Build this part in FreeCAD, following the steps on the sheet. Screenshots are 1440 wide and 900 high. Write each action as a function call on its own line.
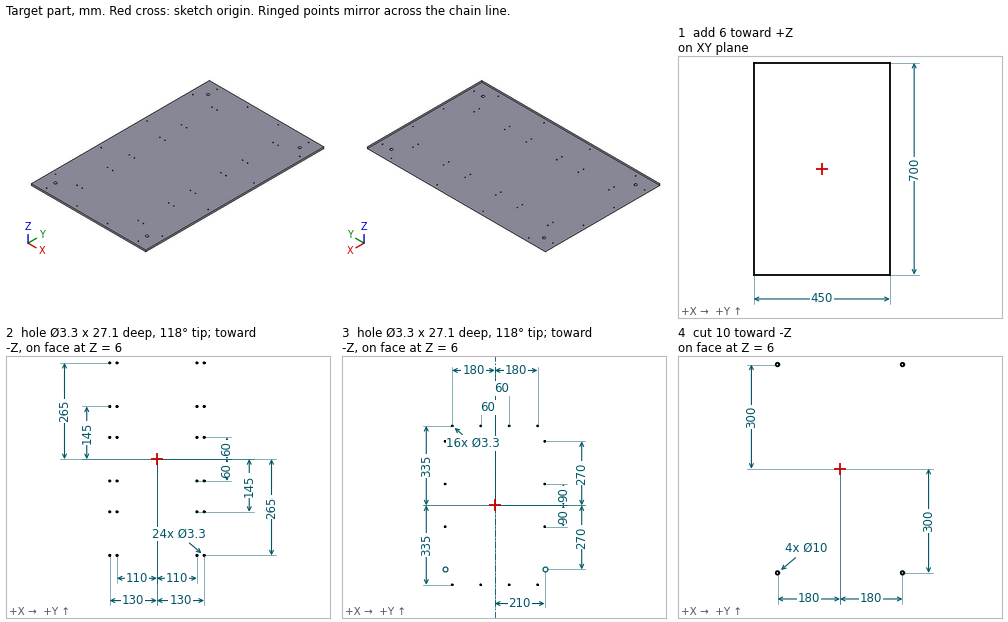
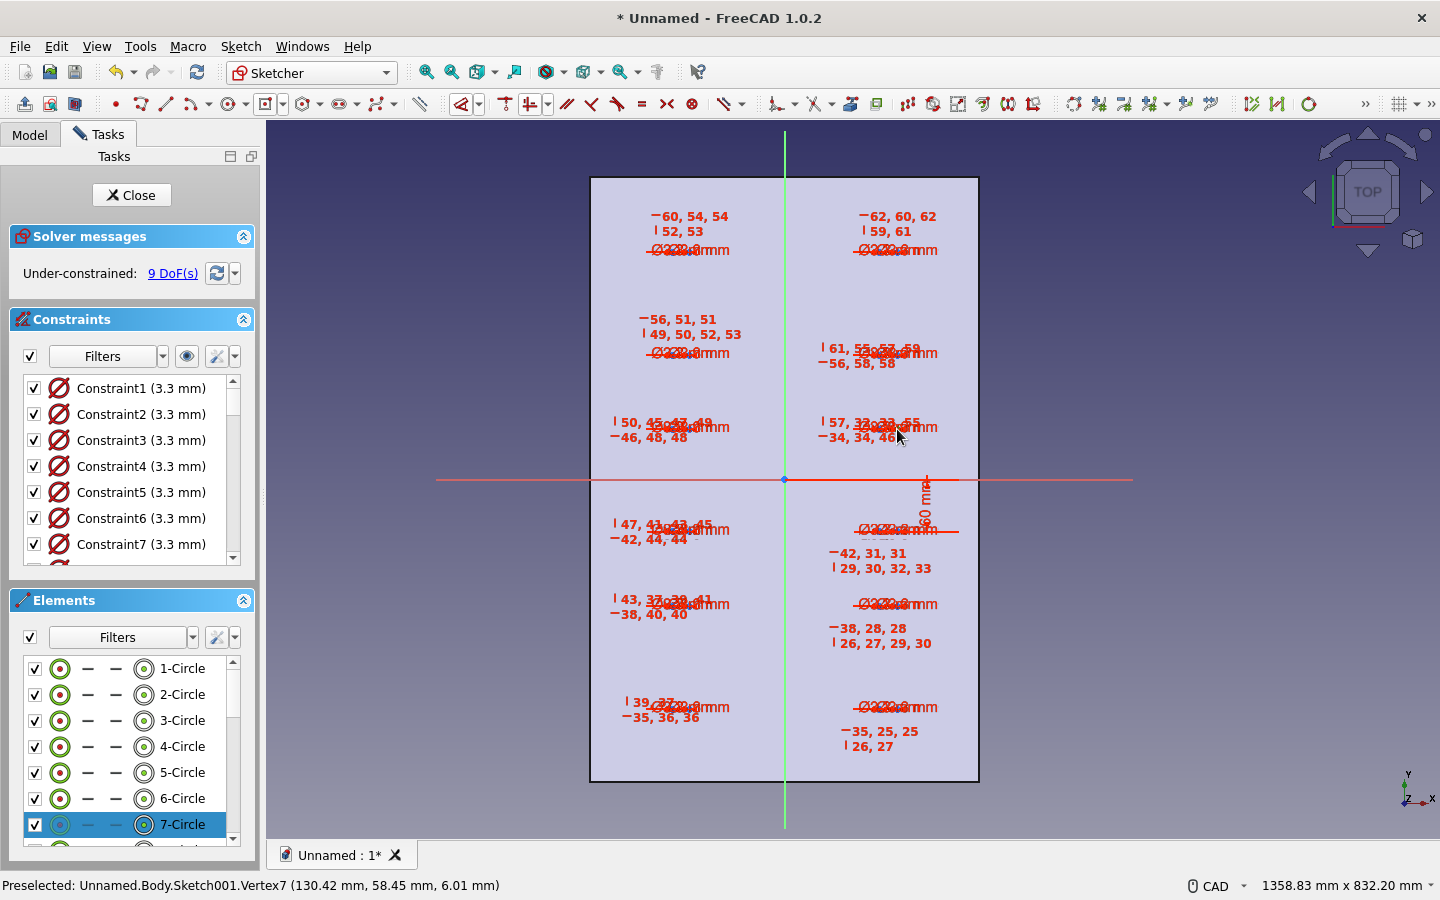
click(478, 104)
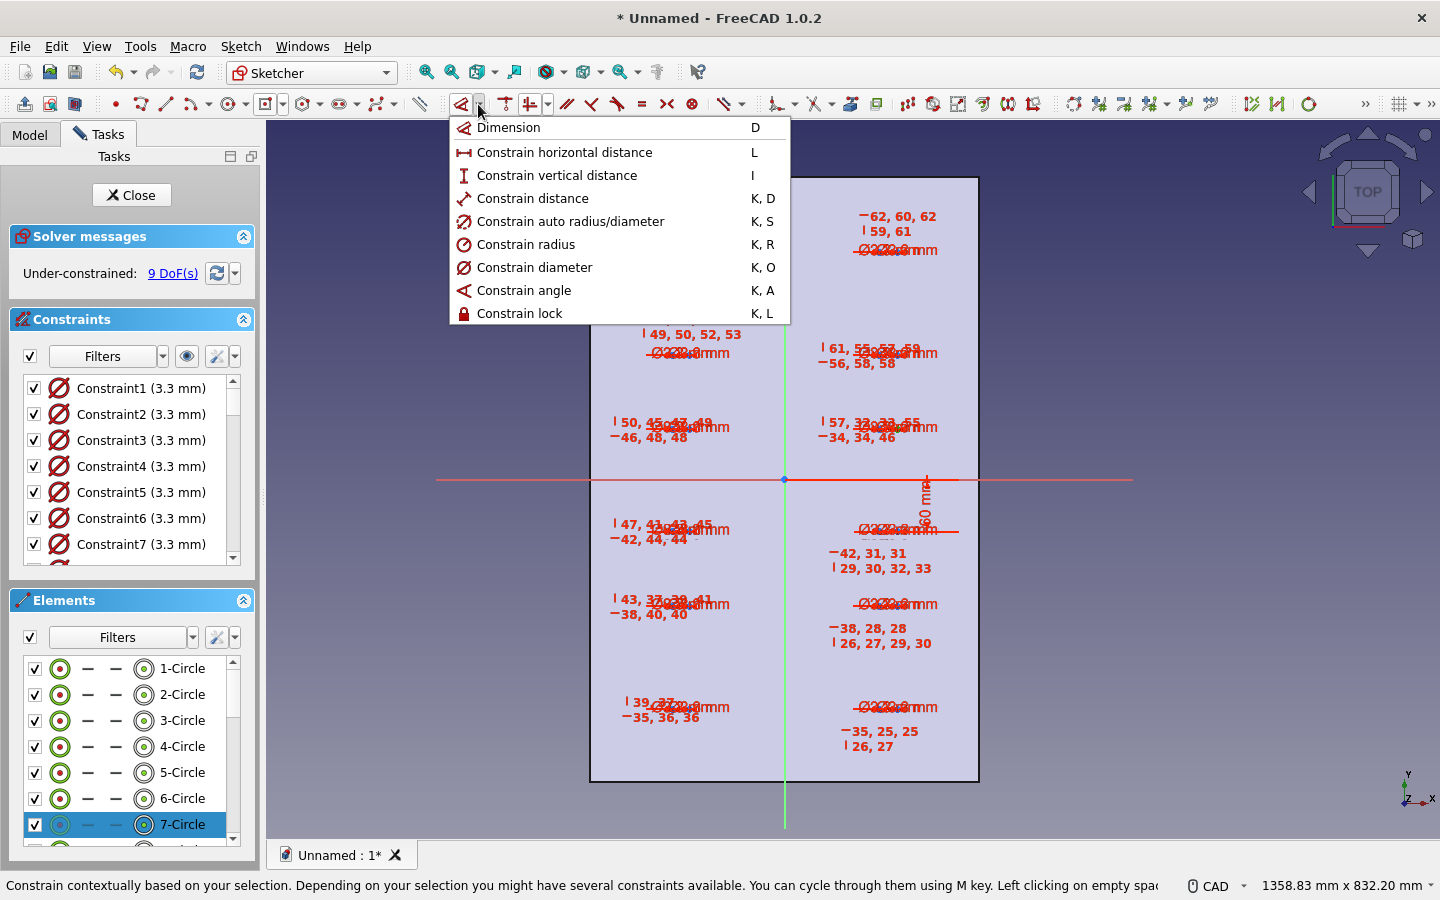
click(620, 176)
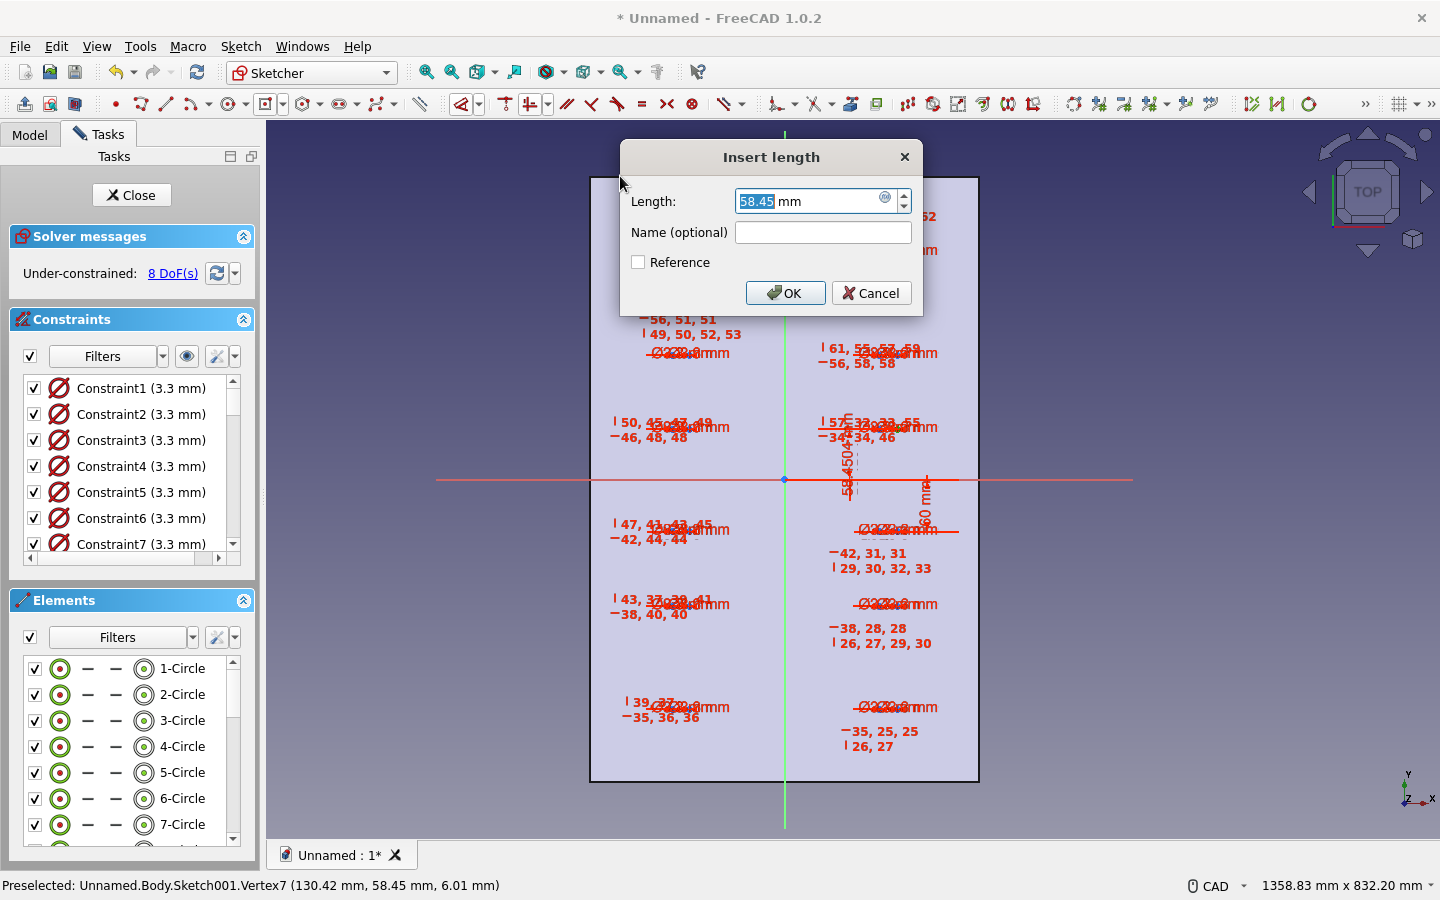
text(60)
key(Return)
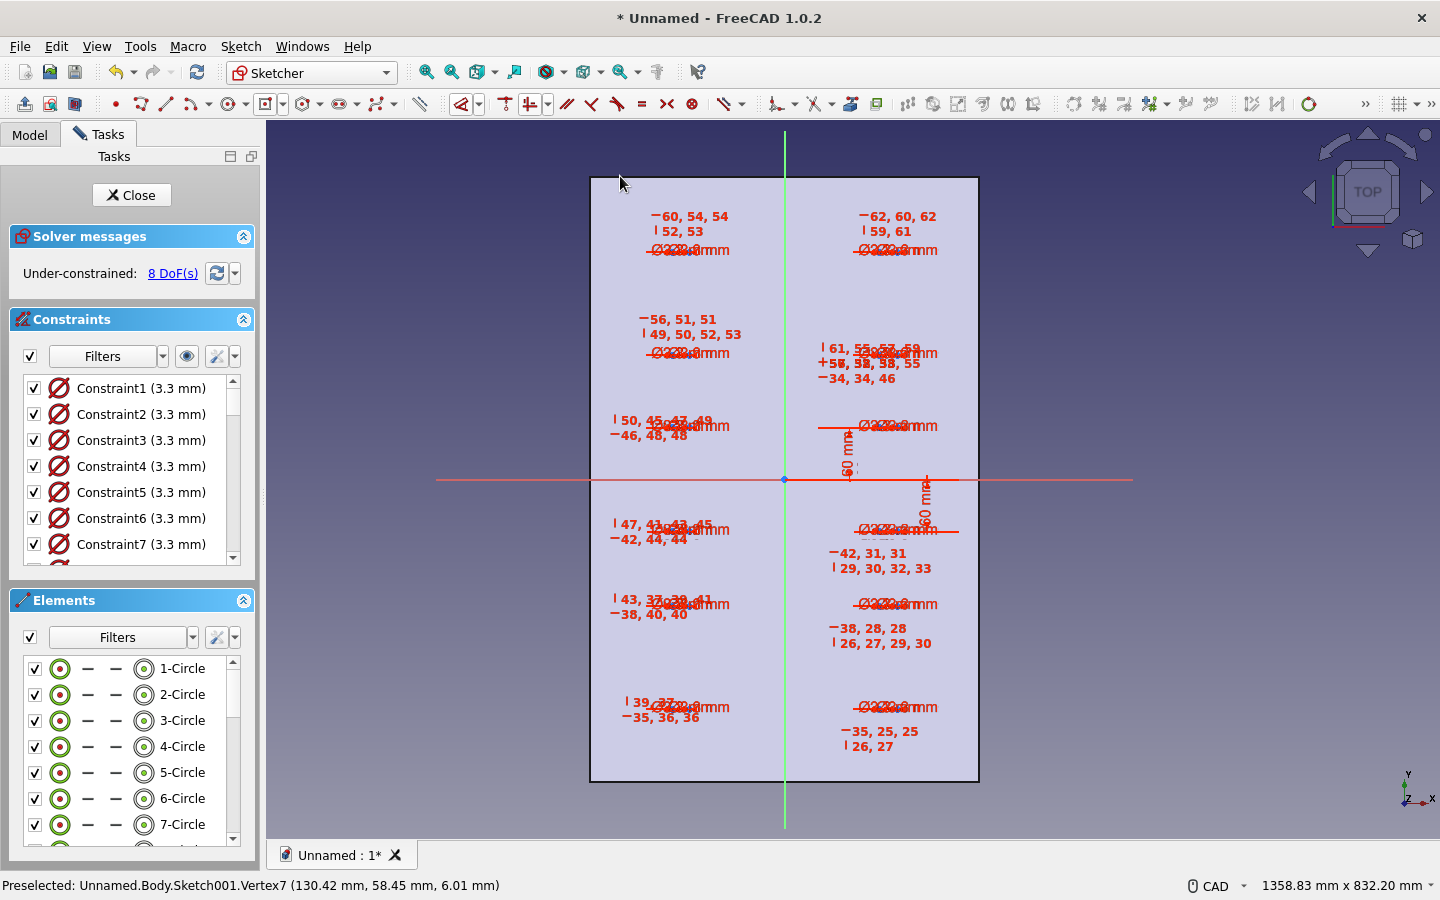
click(897, 709)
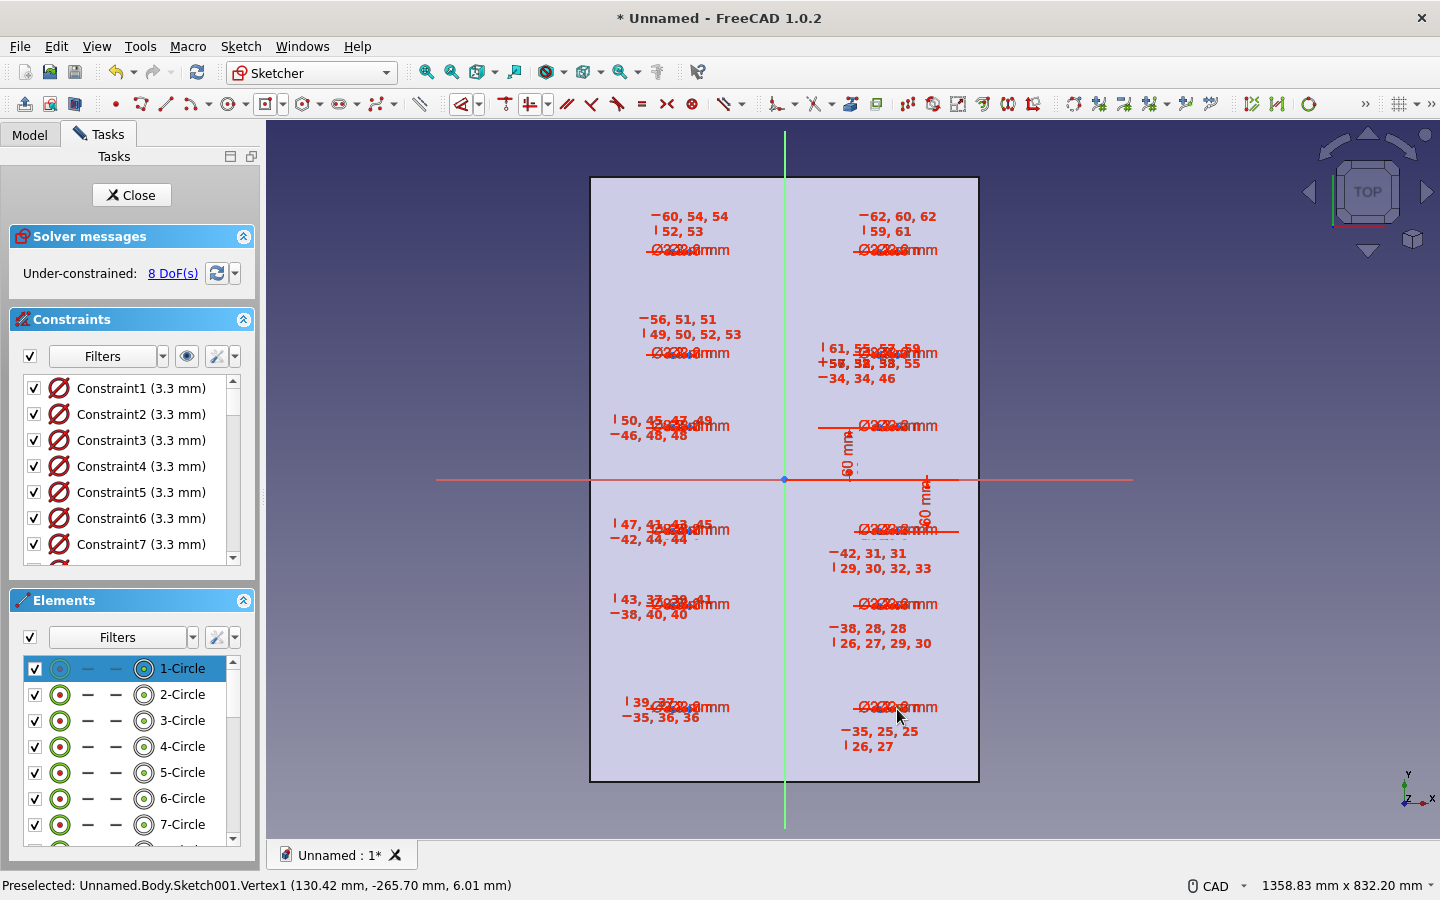
key(l)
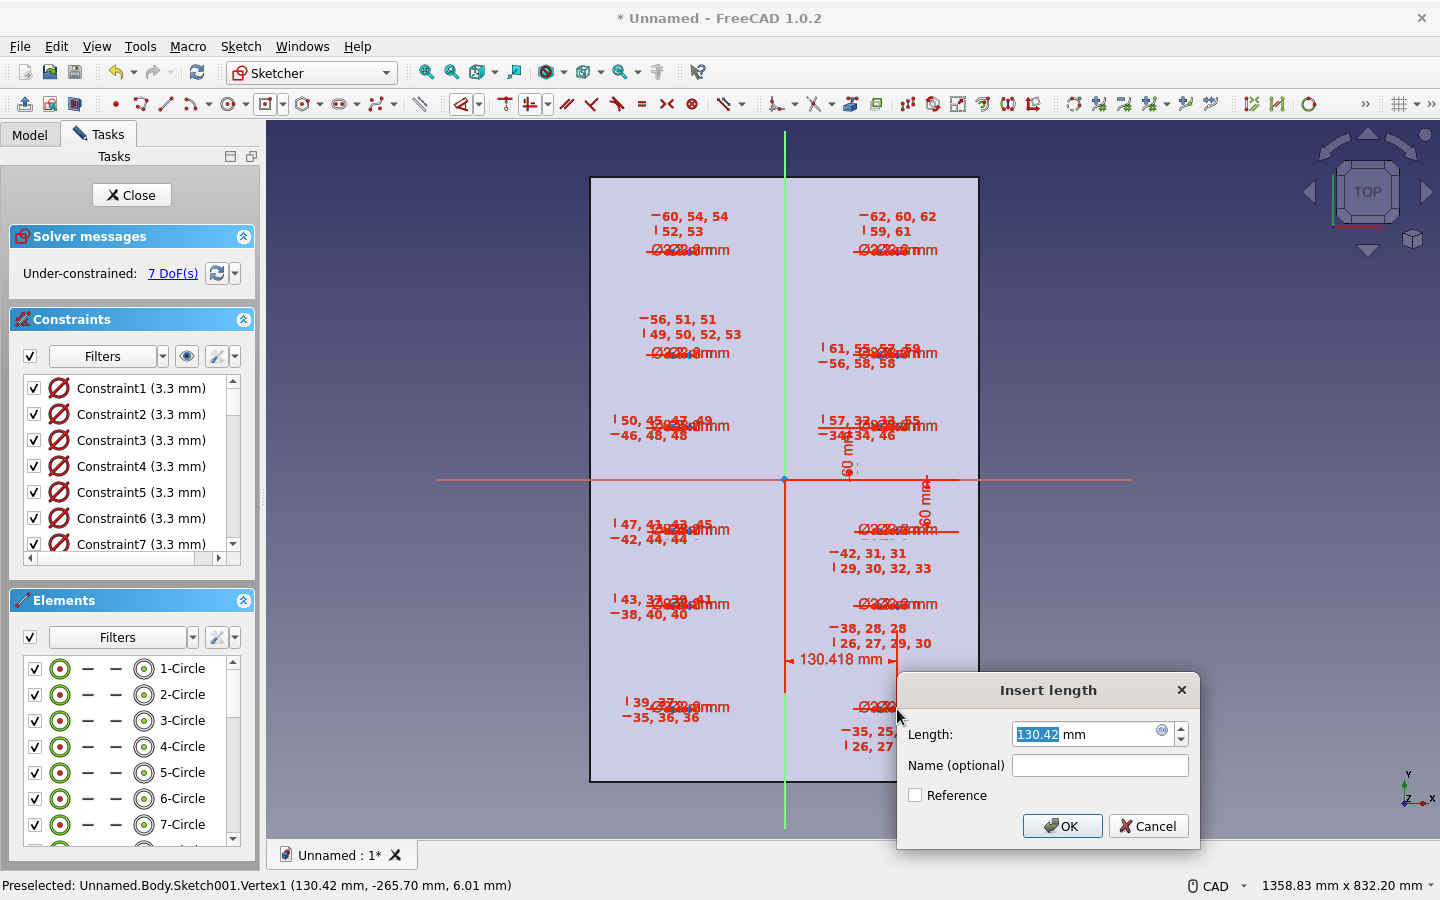
text(130)
key(Return)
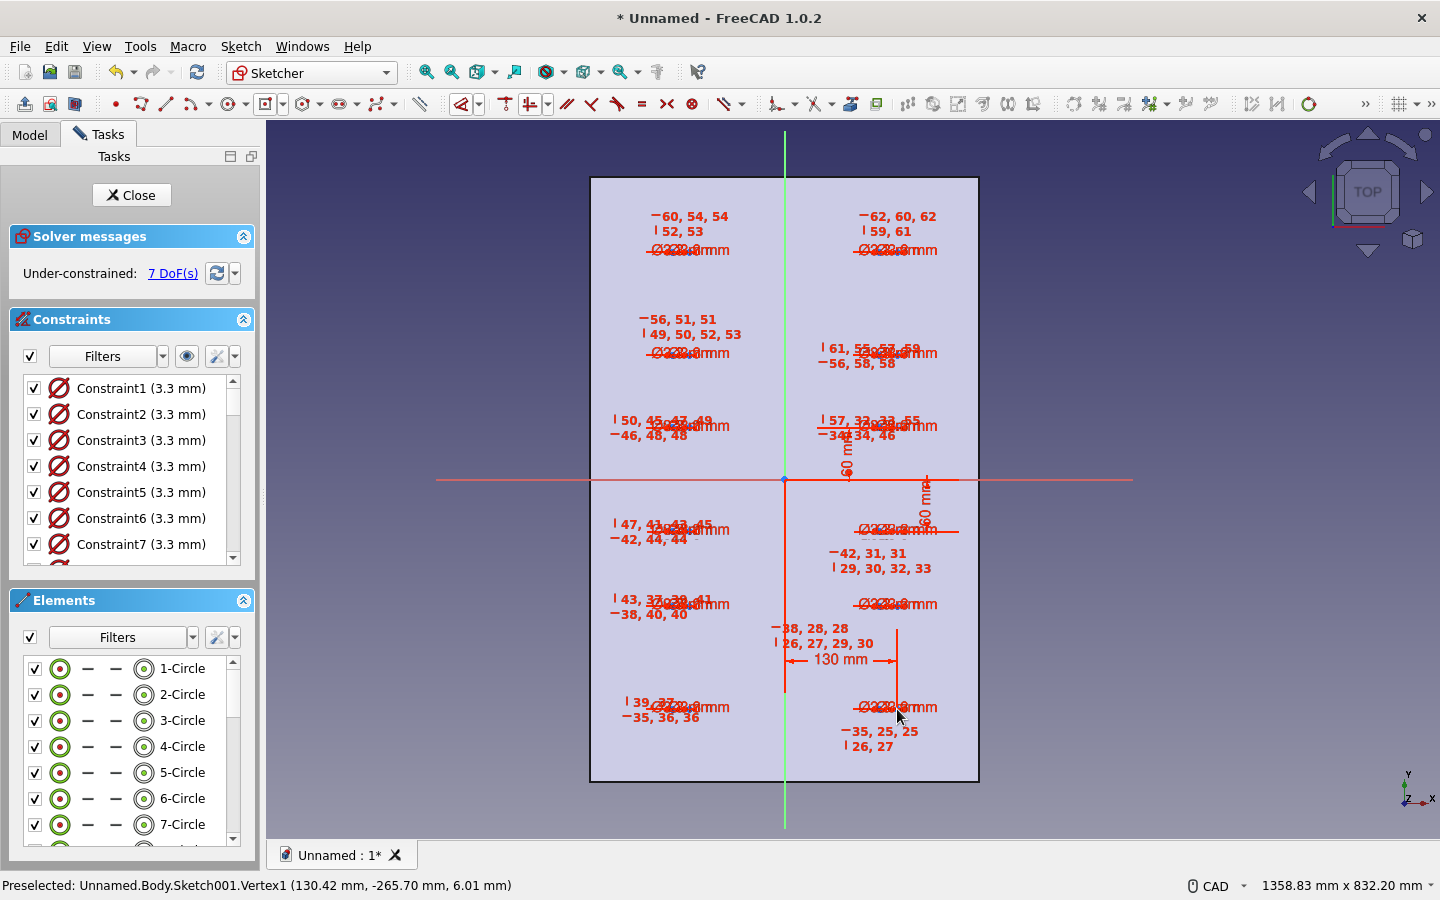
click(897, 709)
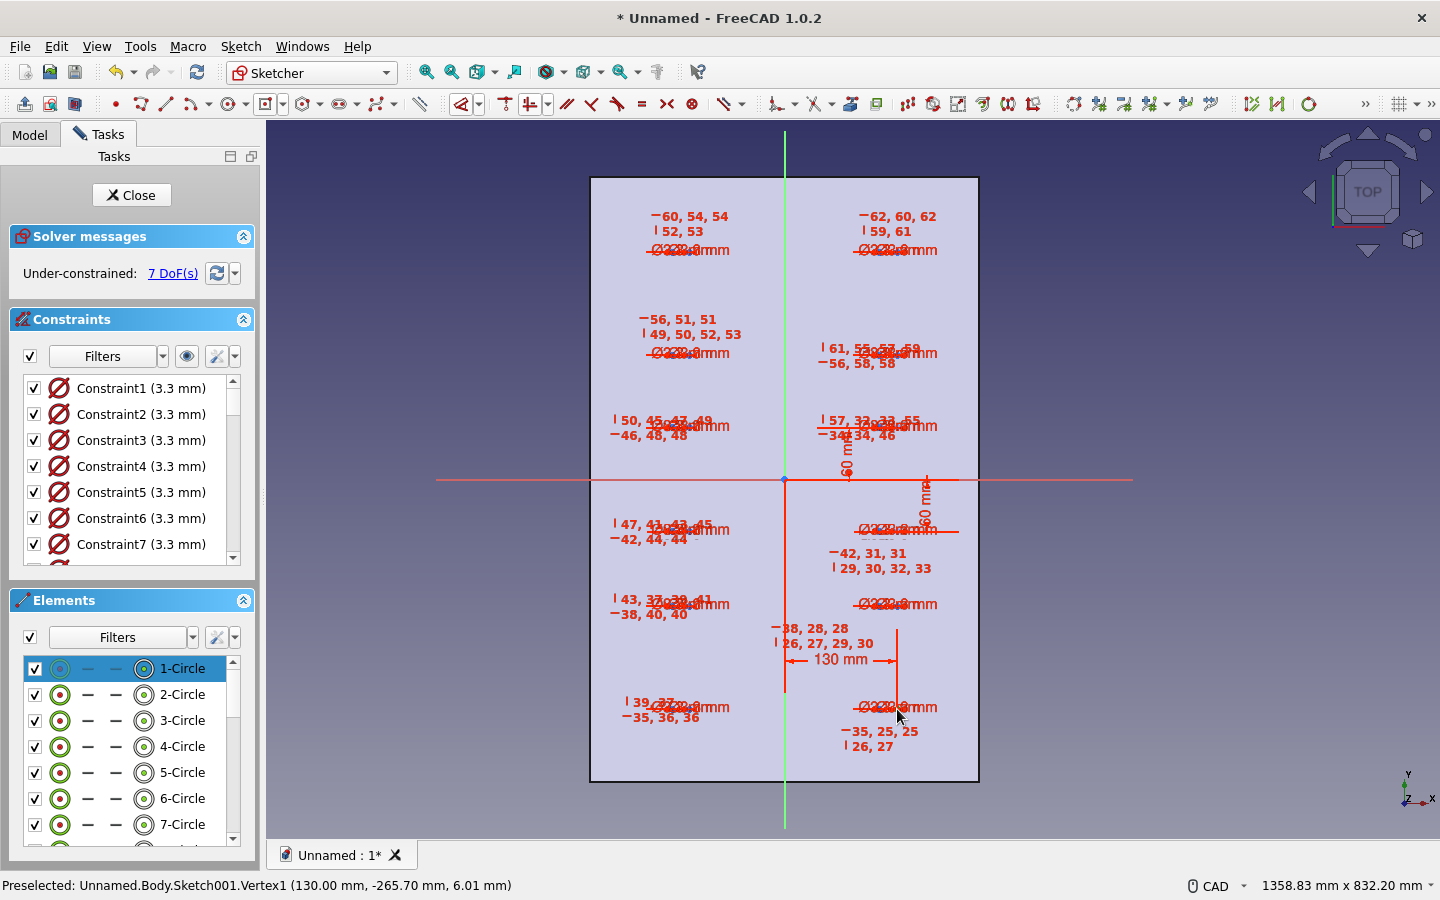
click(478, 104)